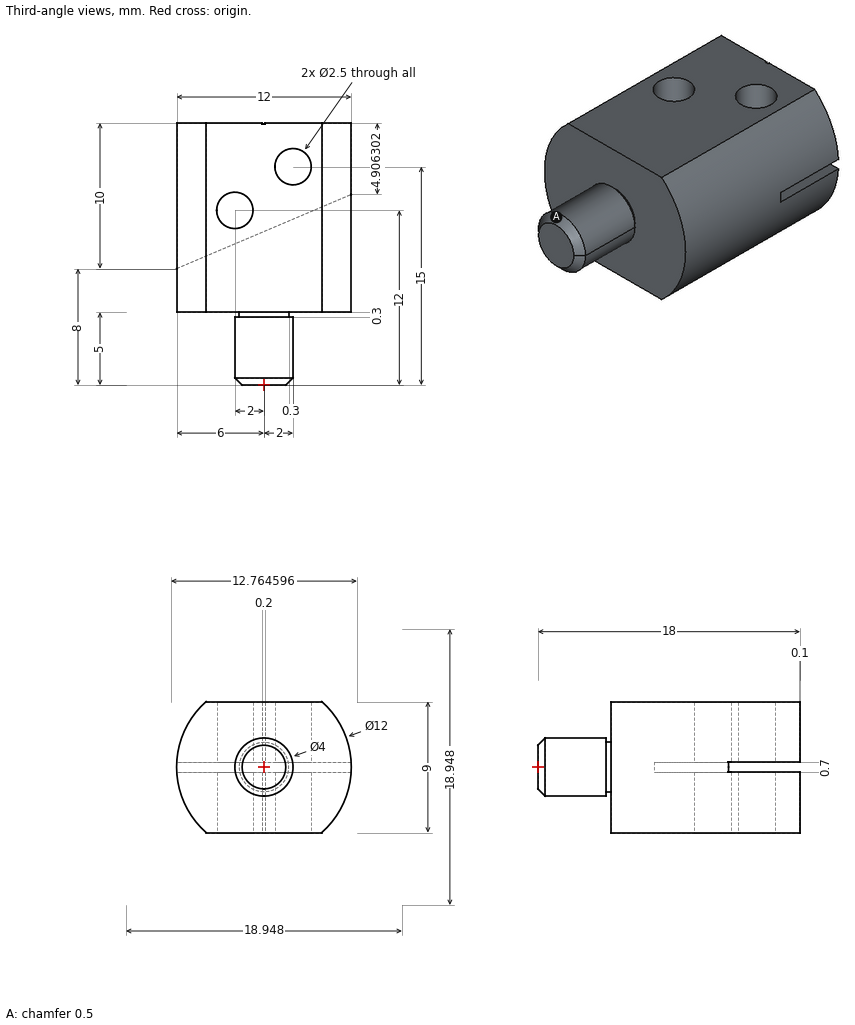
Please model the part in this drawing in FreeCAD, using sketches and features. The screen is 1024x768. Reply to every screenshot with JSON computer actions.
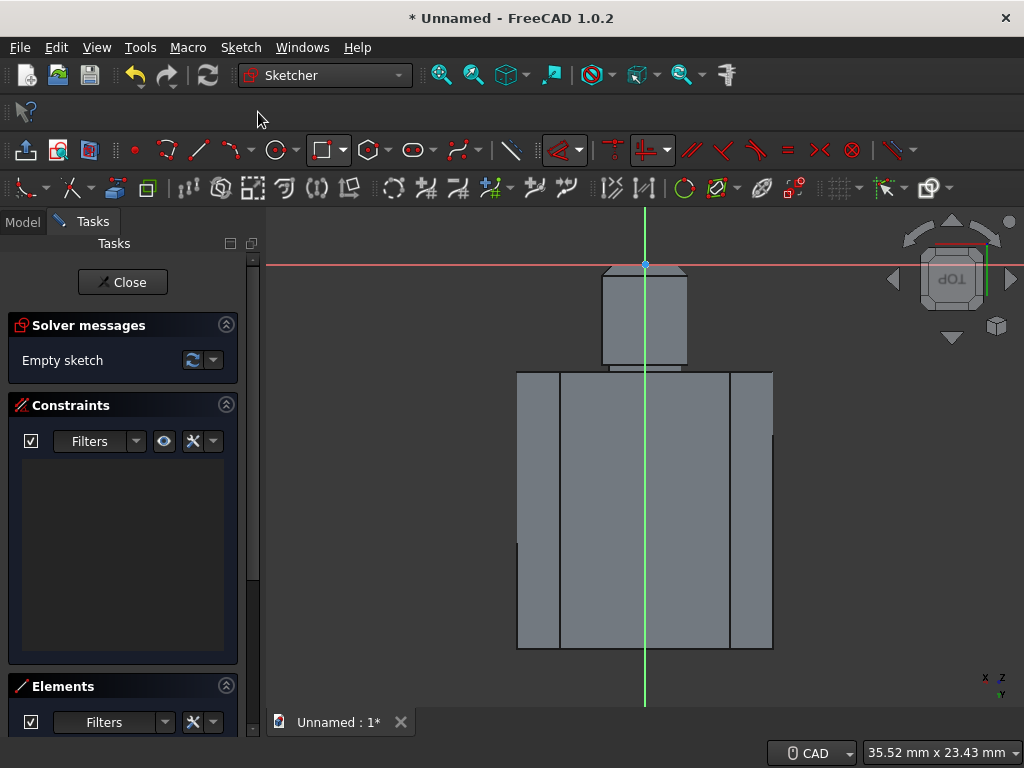
{"action": "scroll", "coordinate": [685, 609], "scroll_direction": "up", "scroll_amount": 5}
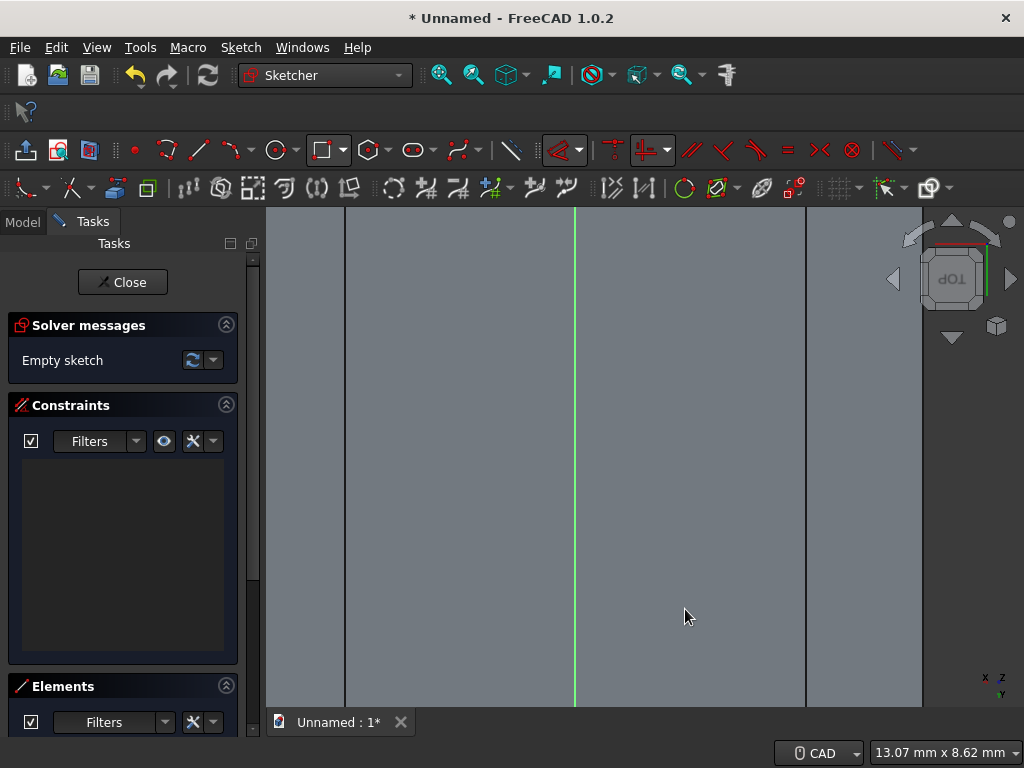
{"action": "left_click", "coordinate": [276, 150]}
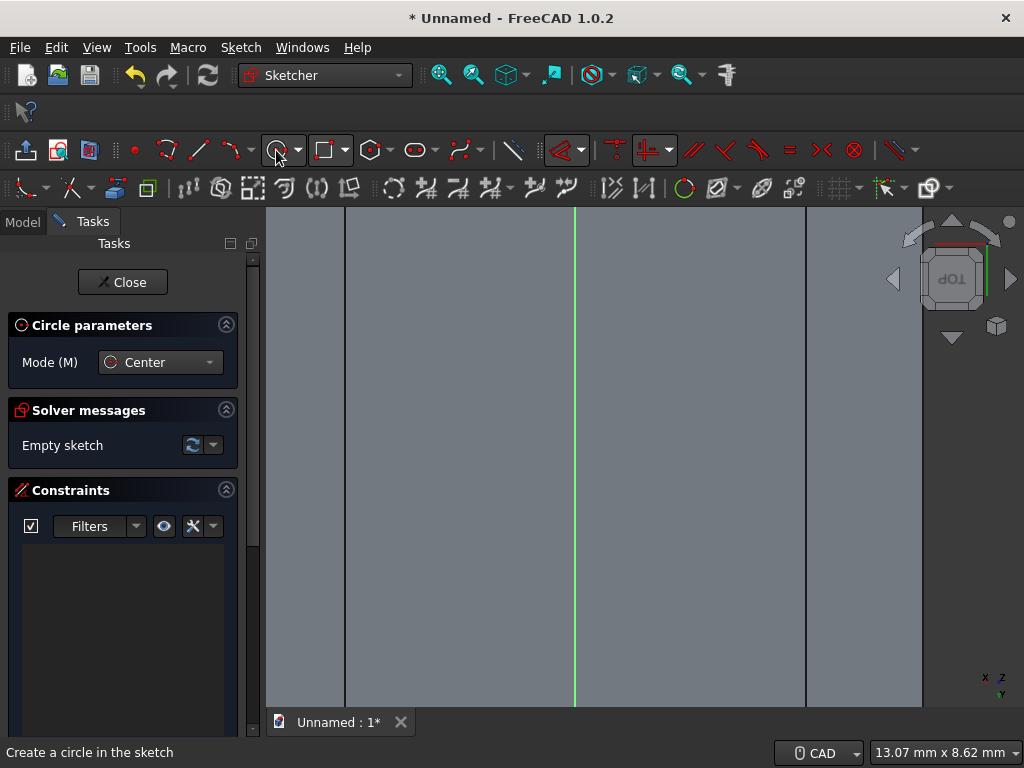
{"action": "left_click", "coordinate": [459, 542]}
{"action": "left_click", "coordinate": [511, 491]}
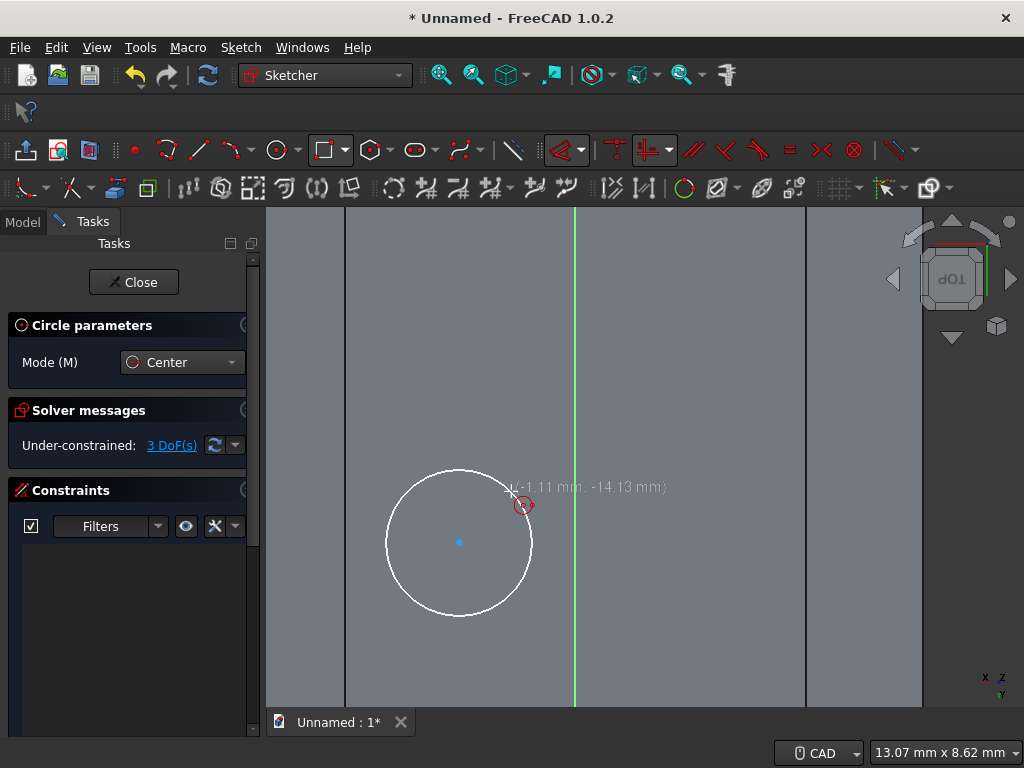
{"action": "left_click", "coordinate": [691, 368]}
{"action": "left_click", "coordinate": [743, 317]}
{"action": "key", "text": "Escape"}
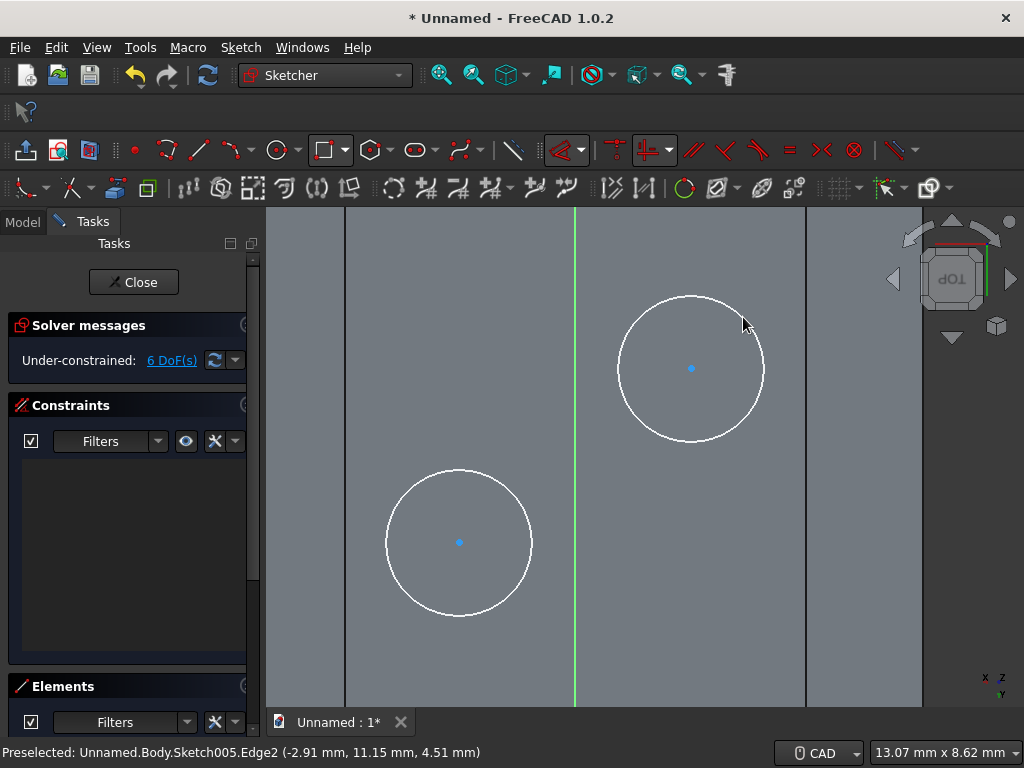
{"action": "left_click", "coordinate": [510, 491]}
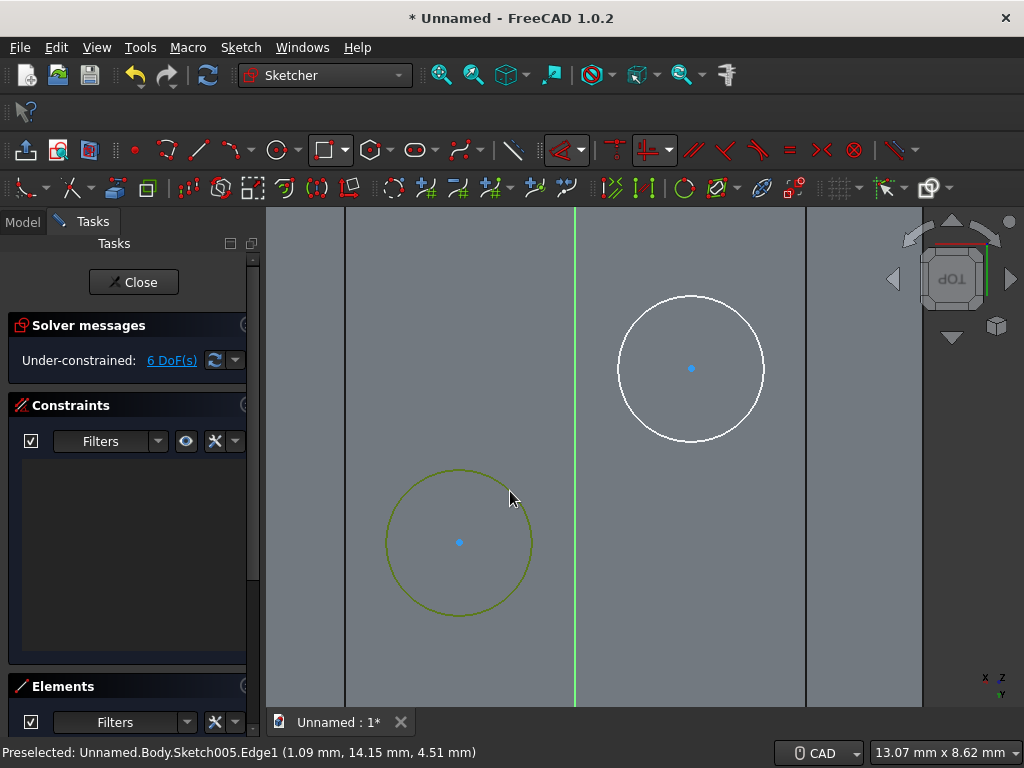
{"action": "left_click", "coordinate": [742, 317]}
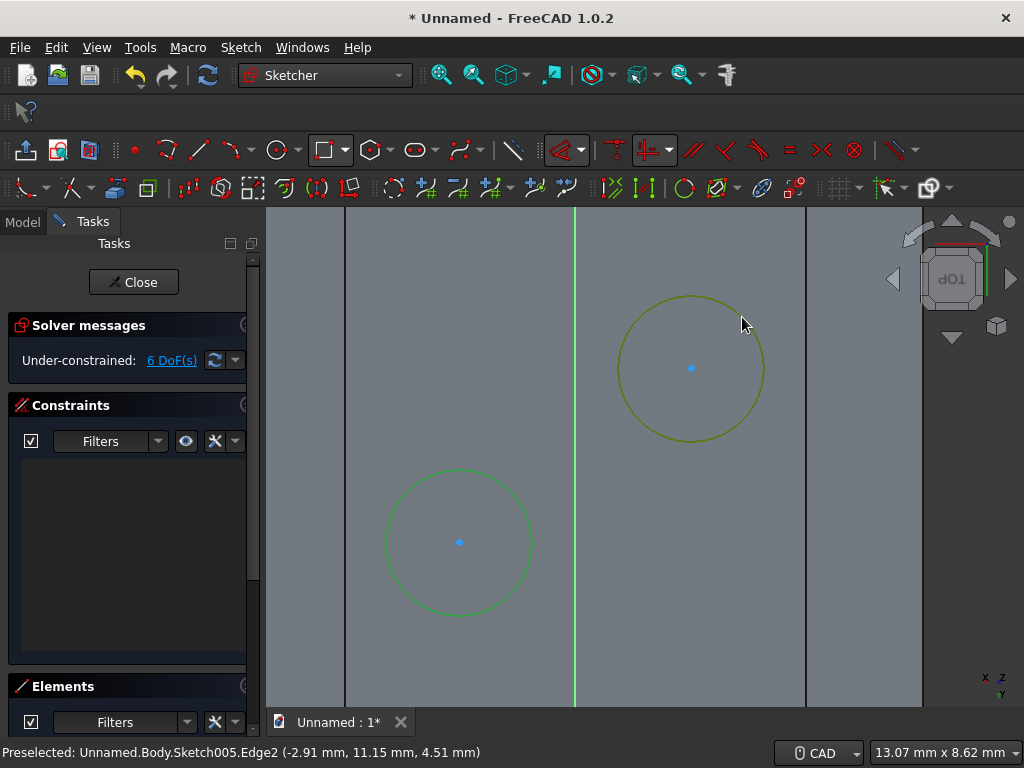
{"action": "left_click", "coordinate": [790, 150]}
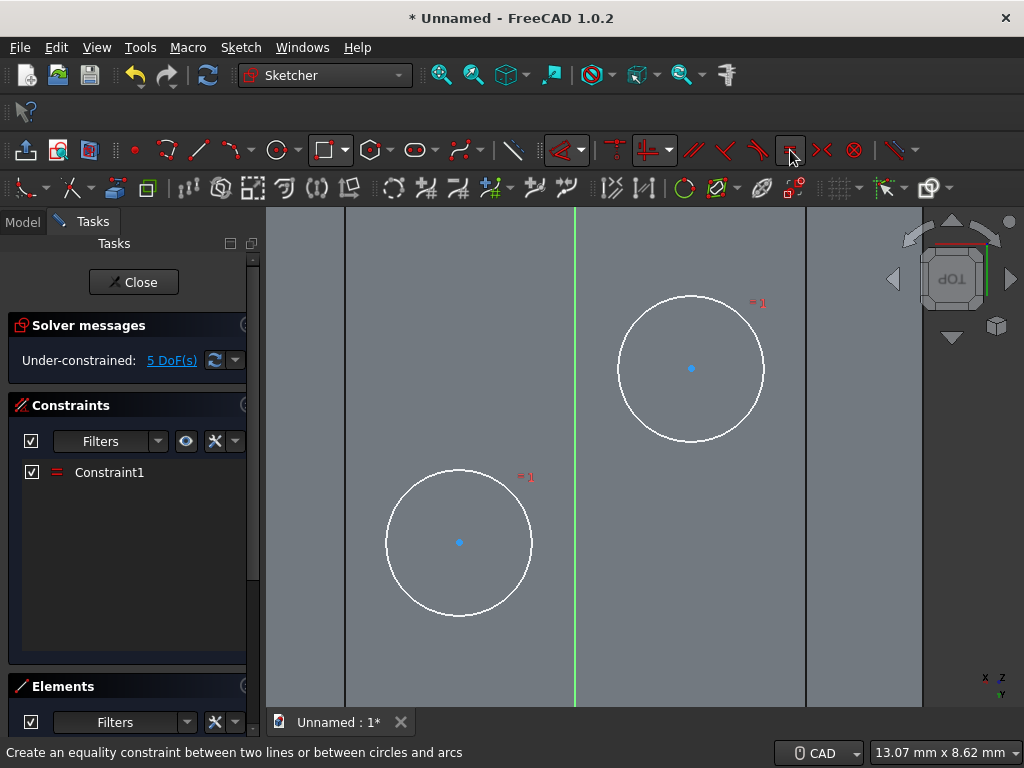
{"action": "left_click", "coordinate": [510, 491]}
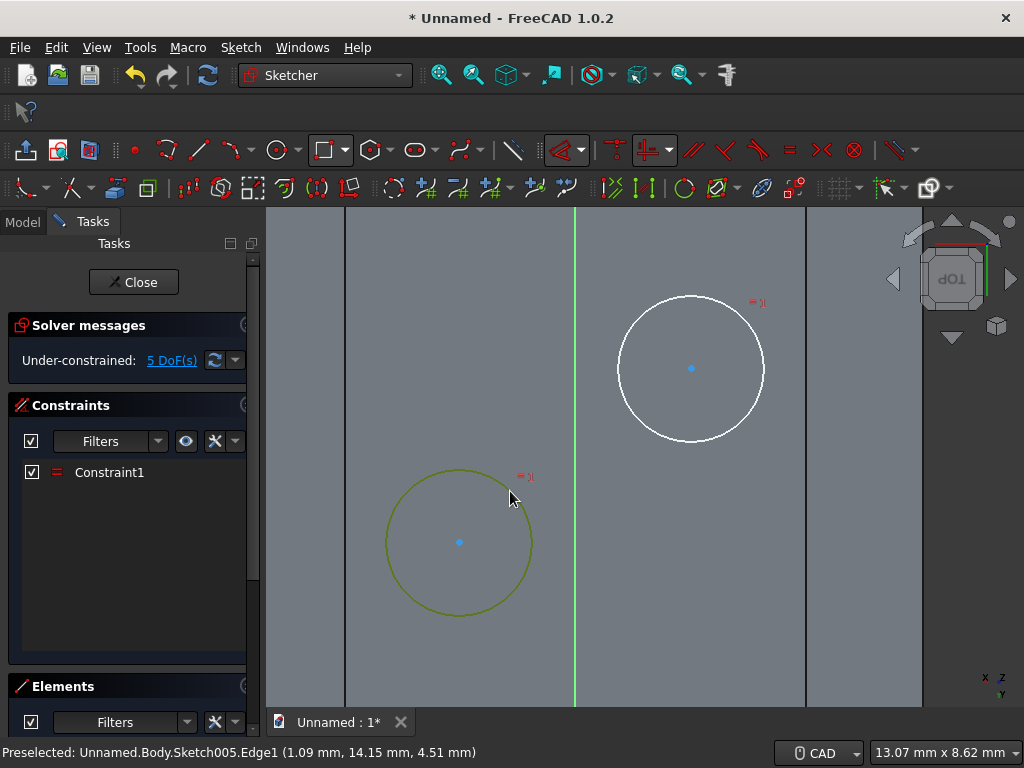
{"action": "left_click", "coordinate": [584, 150]}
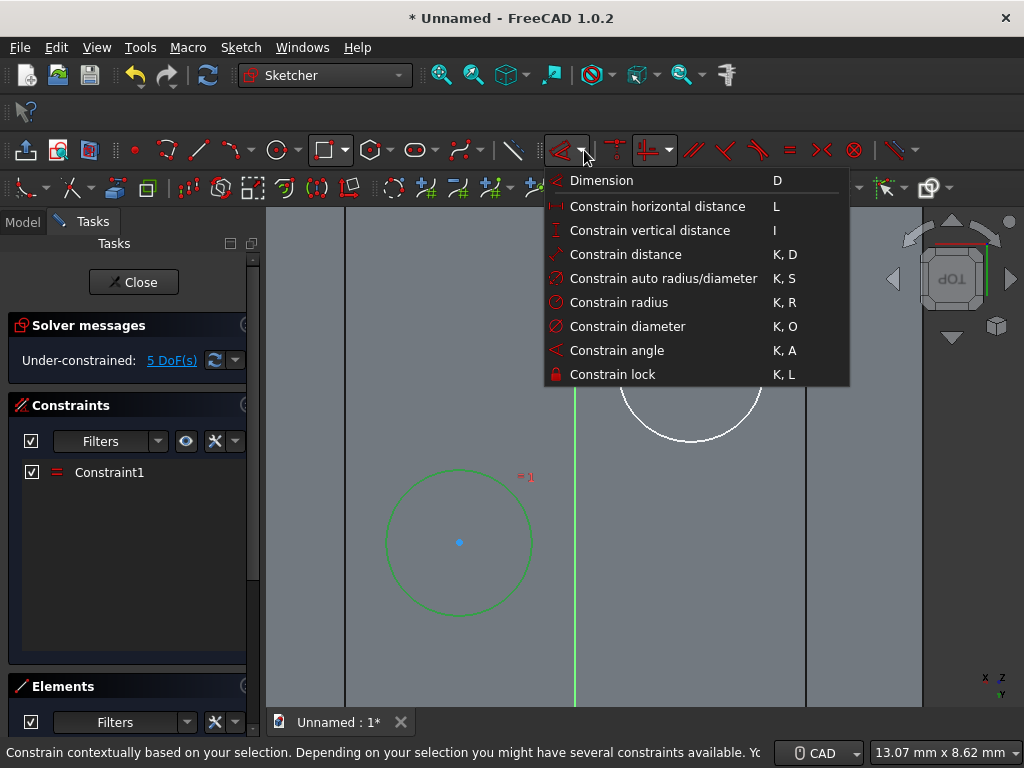
{"action": "left_click", "coordinate": [697, 326]}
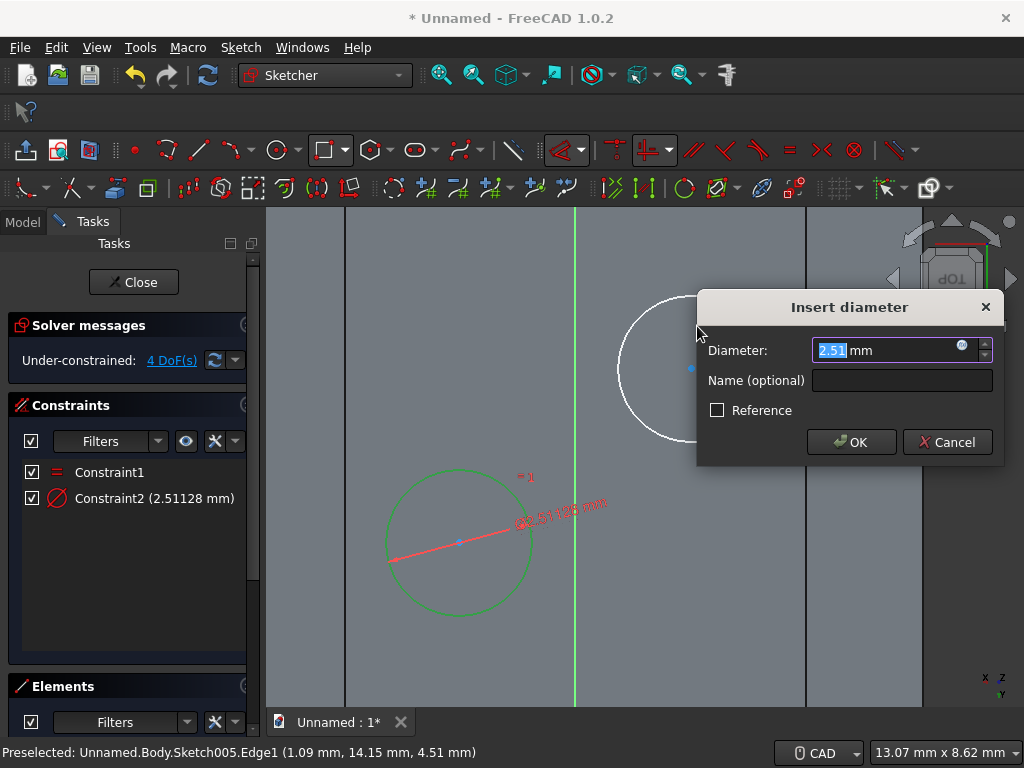
{"action": "type", "text": "2.5"}
{"action": "key", "text": "Return"}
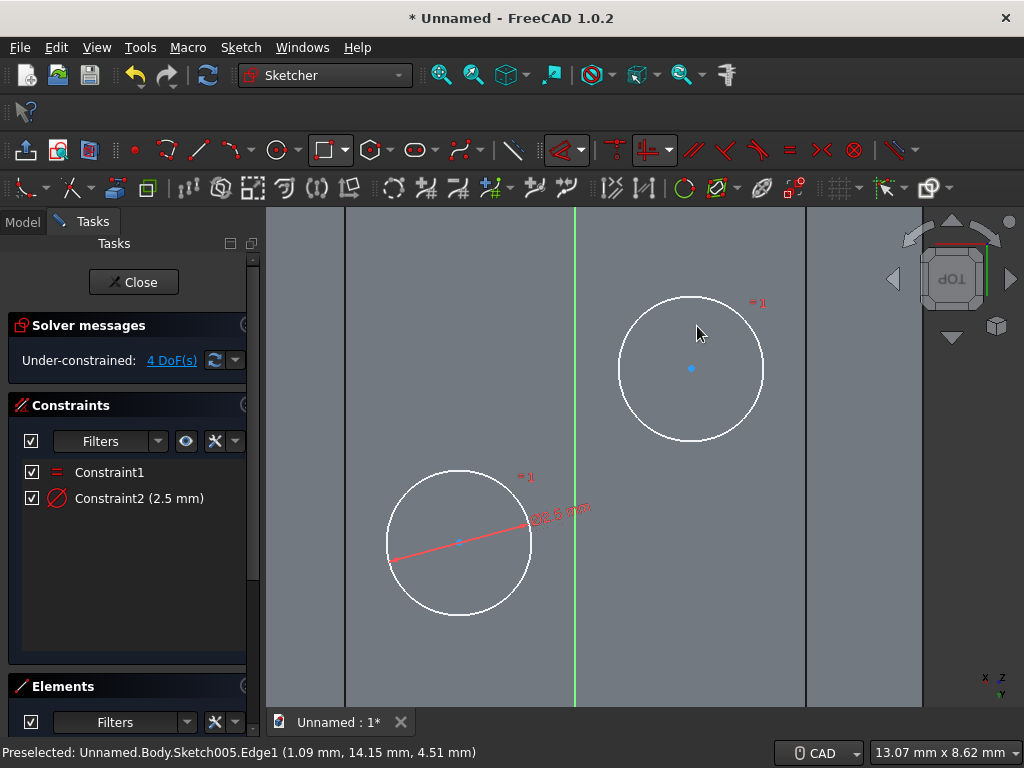
{"action": "left_click", "coordinate": [459, 543]}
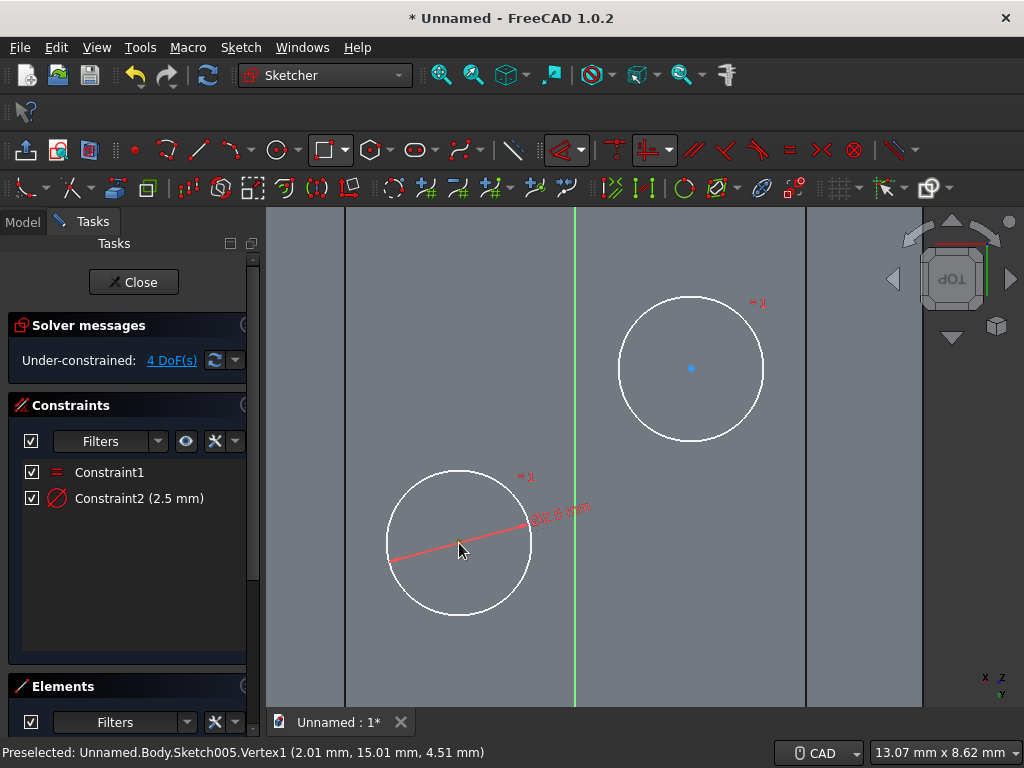
{"action": "key", "text": "l"}